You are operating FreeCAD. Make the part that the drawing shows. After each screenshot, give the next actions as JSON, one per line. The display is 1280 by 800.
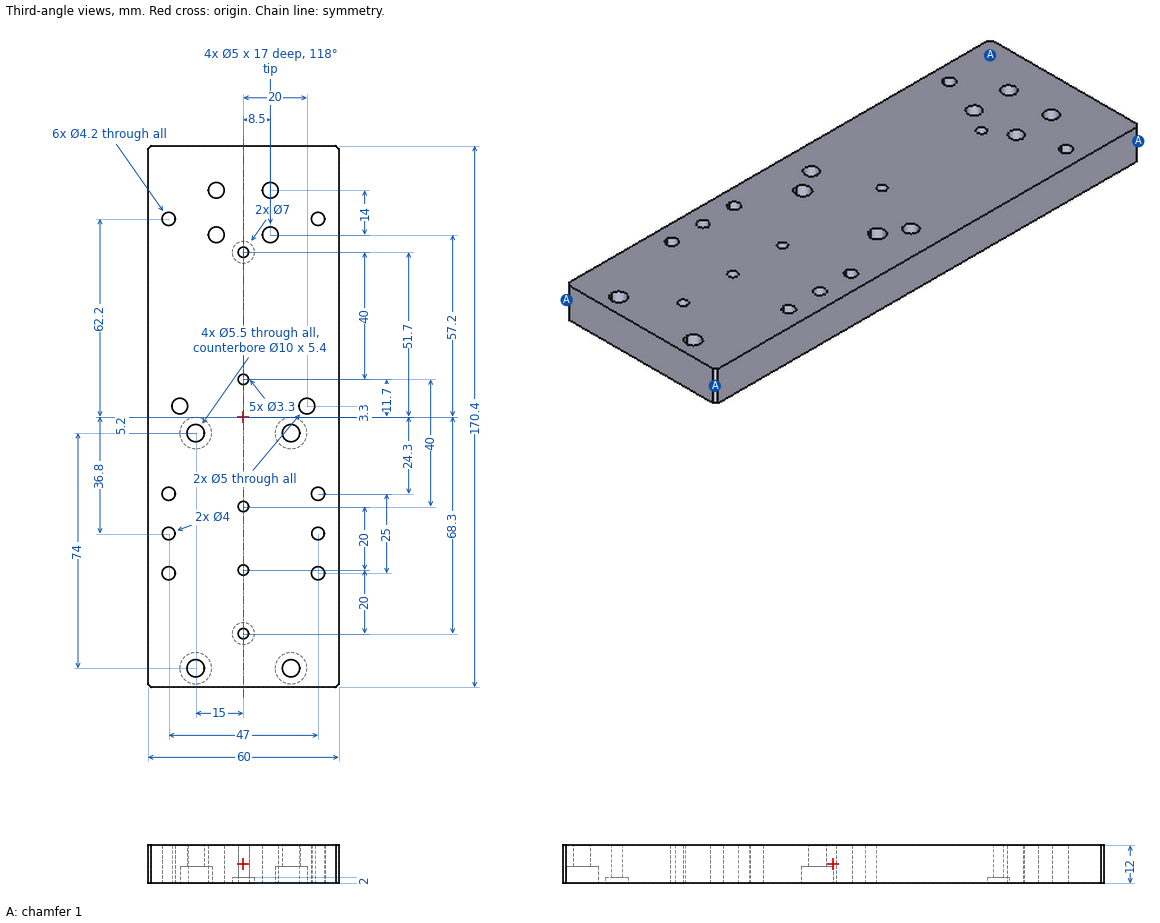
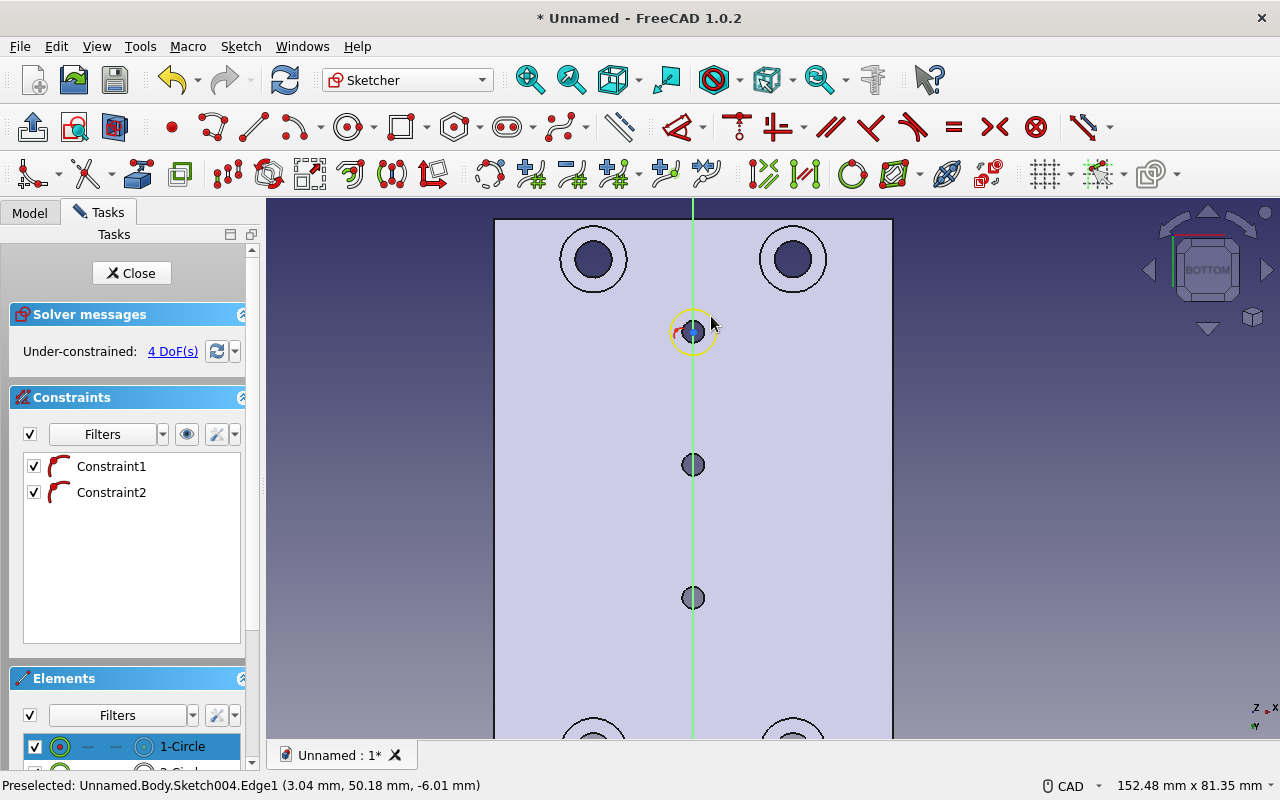
{"action": "left_click", "coordinate": [709, 316]}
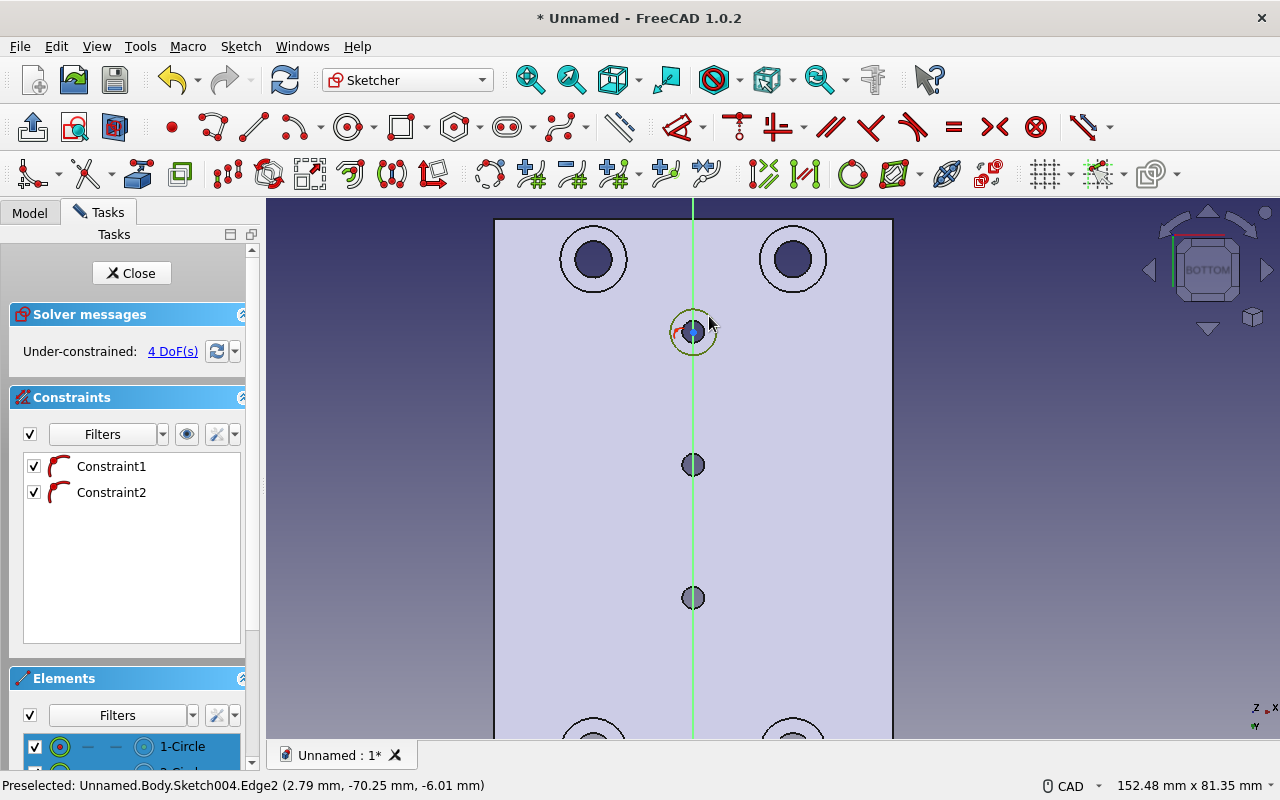
{"action": "key", "text": "e"}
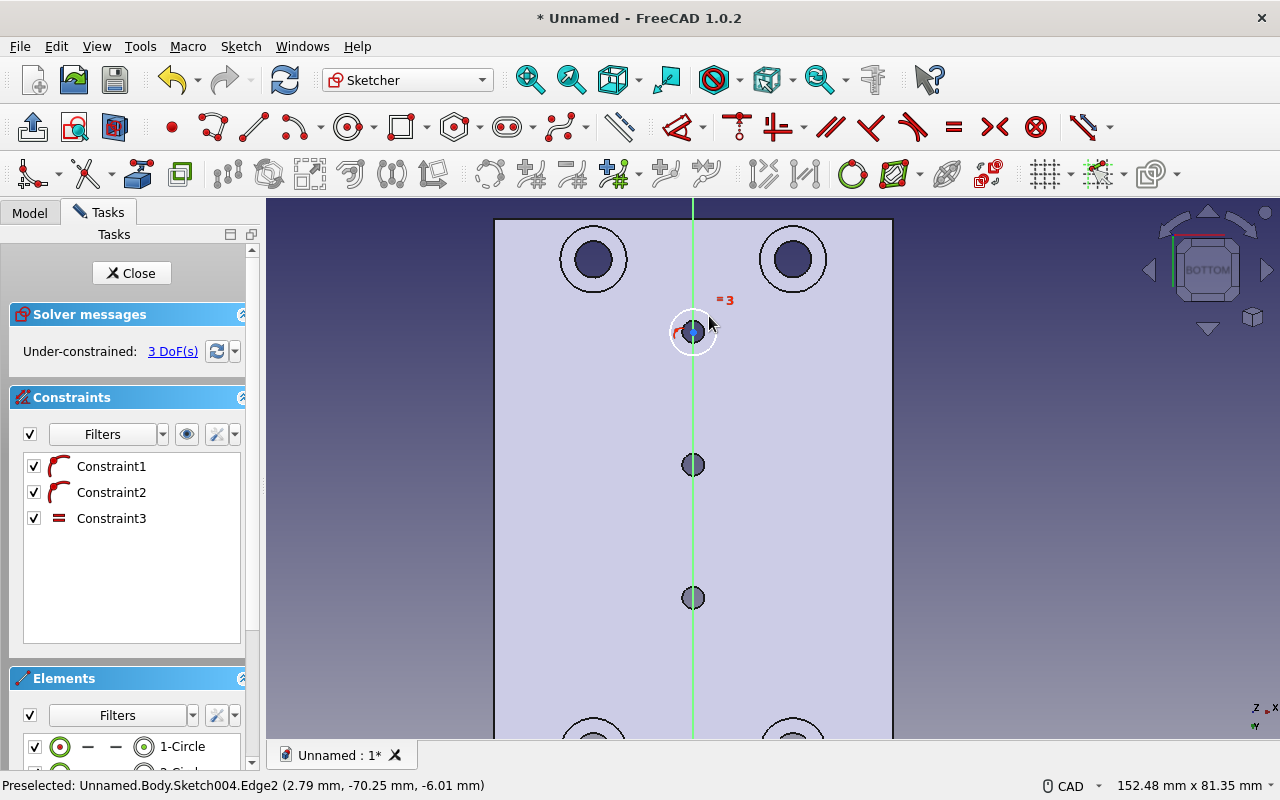
{"action": "left_click", "coordinate": [676, 128]}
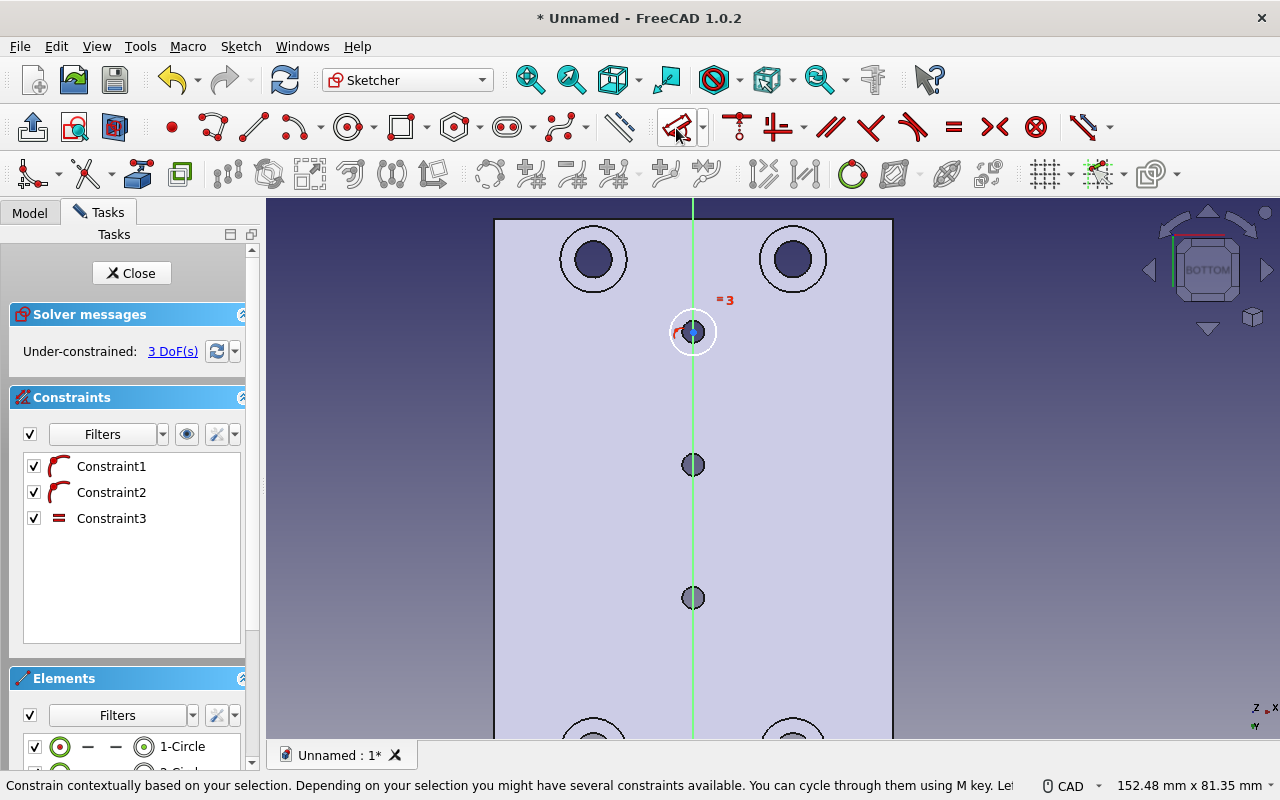
{"action": "scroll", "coordinate": [711, 316], "scroll_direction": "down", "scroll_amount": 5}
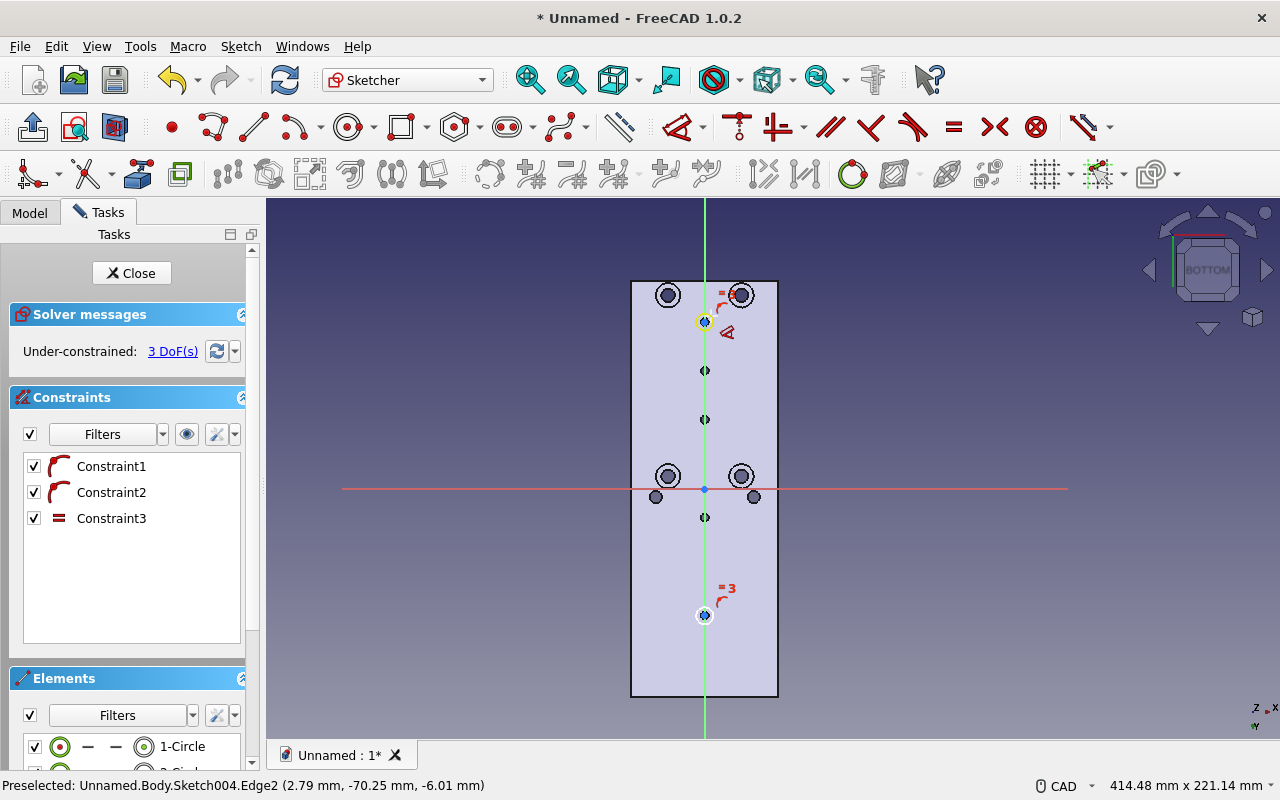
{"action": "scroll", "coordinate": [711, 610], "scroll_direction": "up", "scroll_amount": 5}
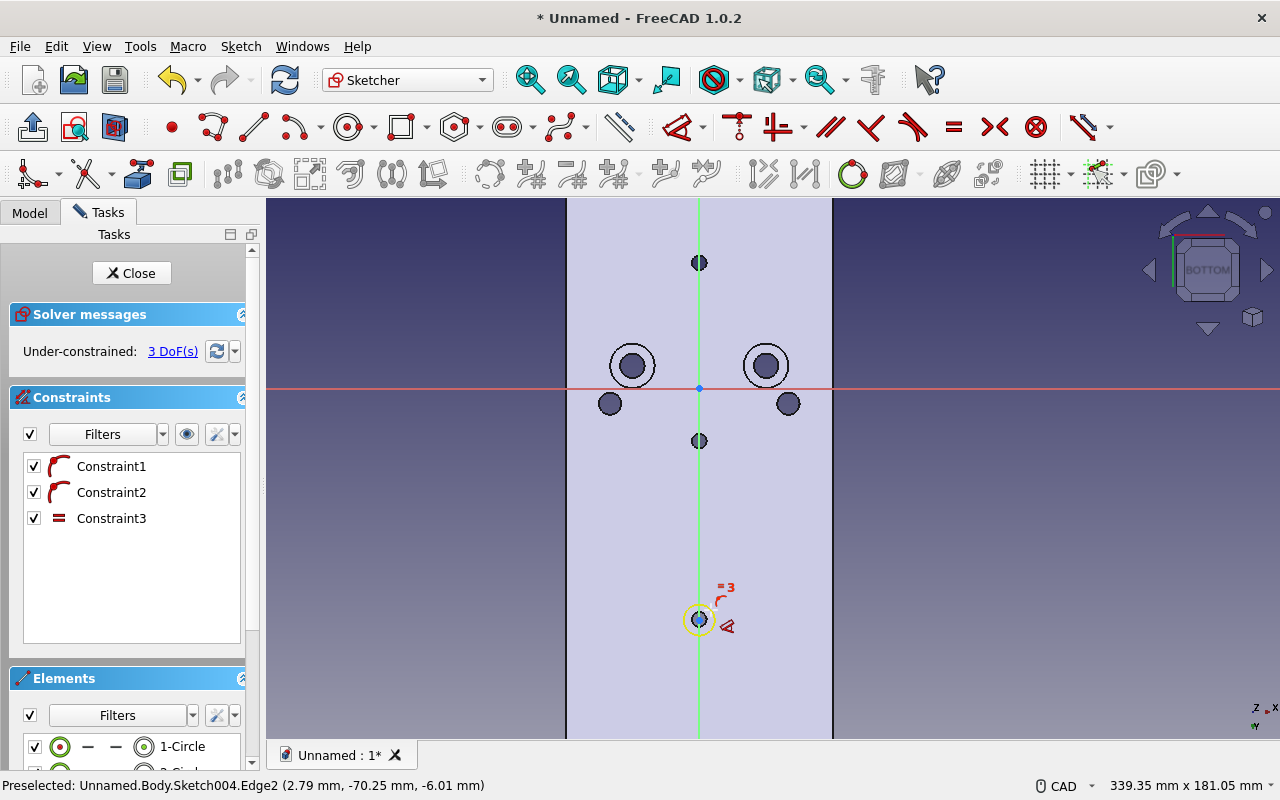
{"action": "left_click", "coordinate": [710, 608]}
{"action": "left_click", "coordinate": [733, 585]}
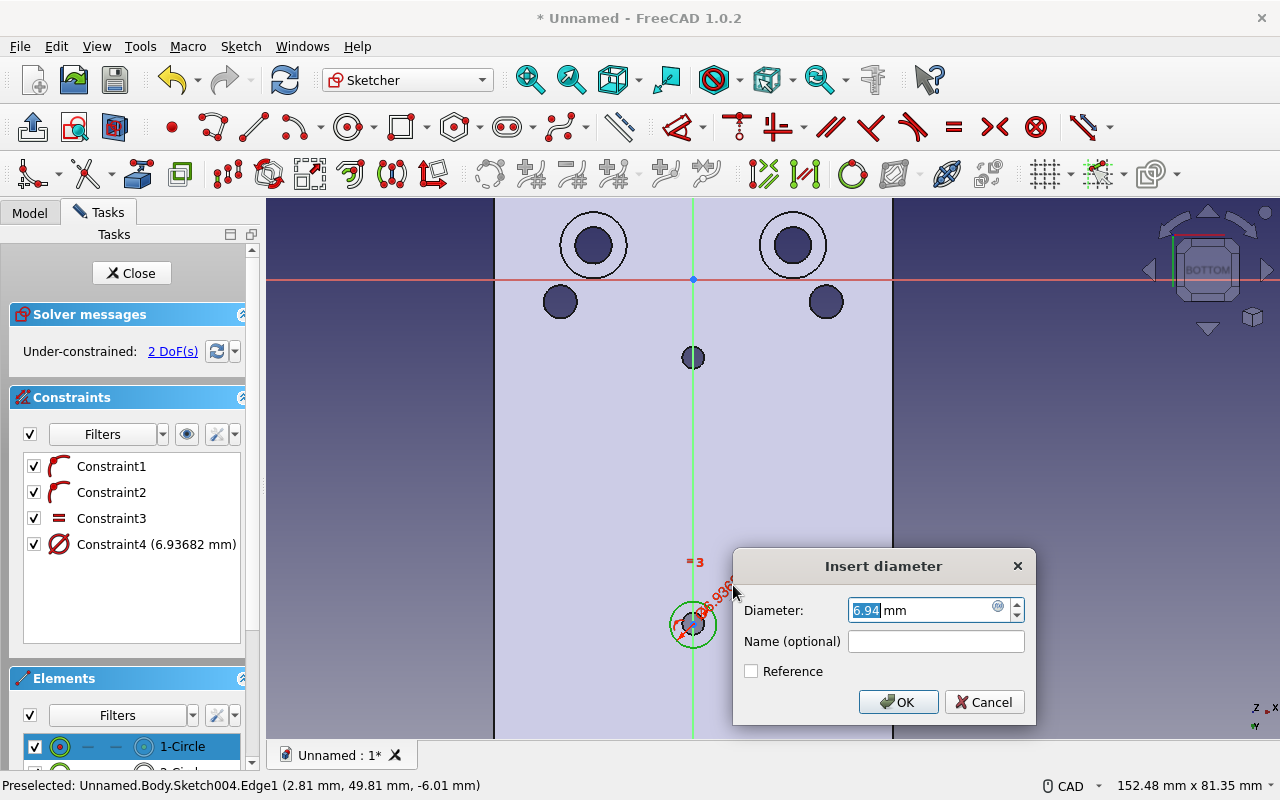
{"action": "type", "text": "7"}
{"action": "key", "text": "Return"}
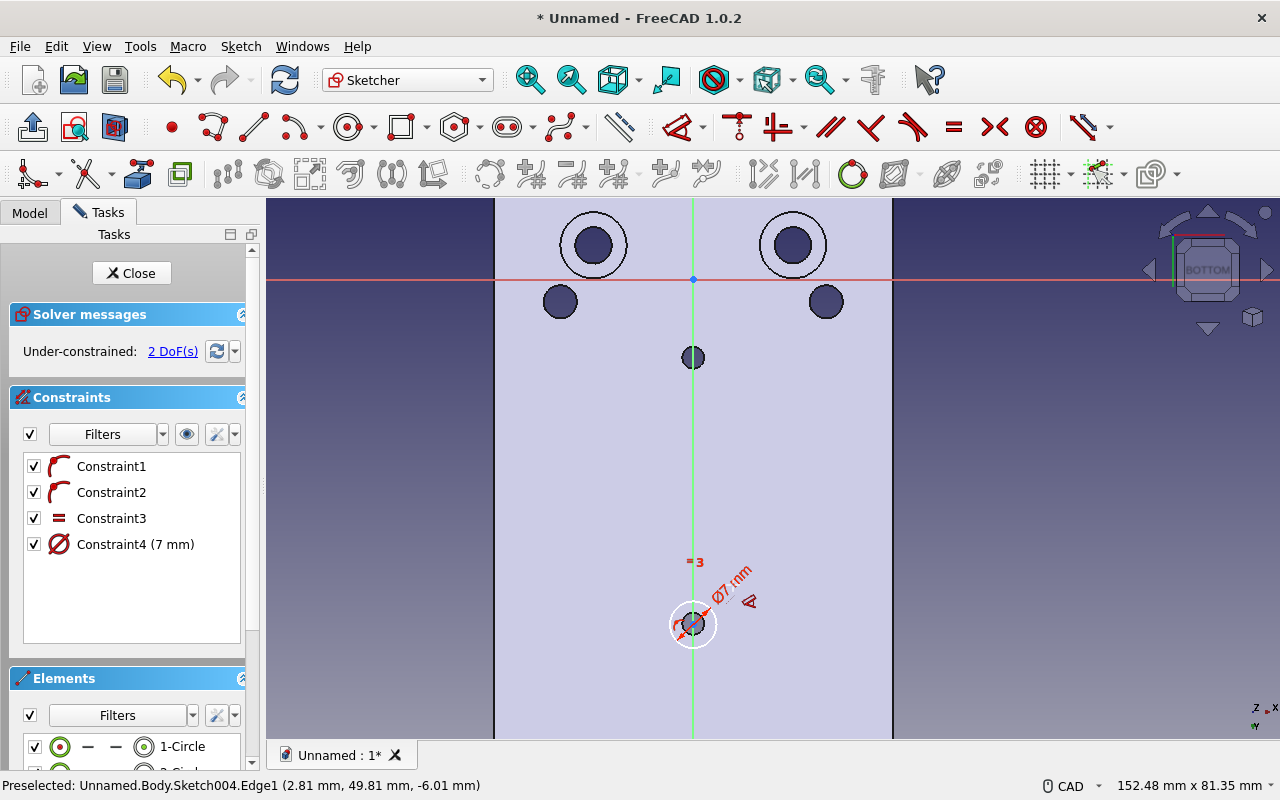
{"action": "left_click", "coordinate": [693, 625]}
{"action": "left_click", "coordinate": [727, 452]}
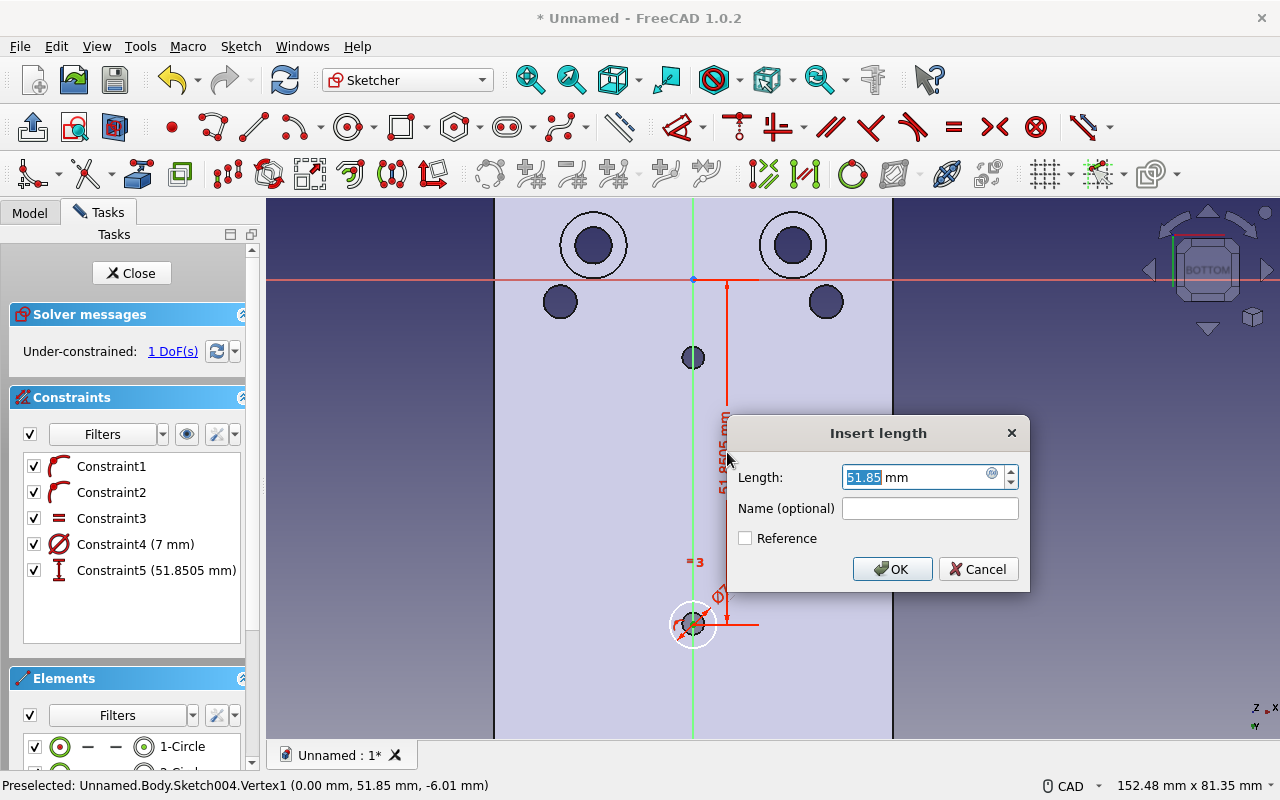
{"action": "type", "text": "51.7"}
{"action": "key", "text": "Return"}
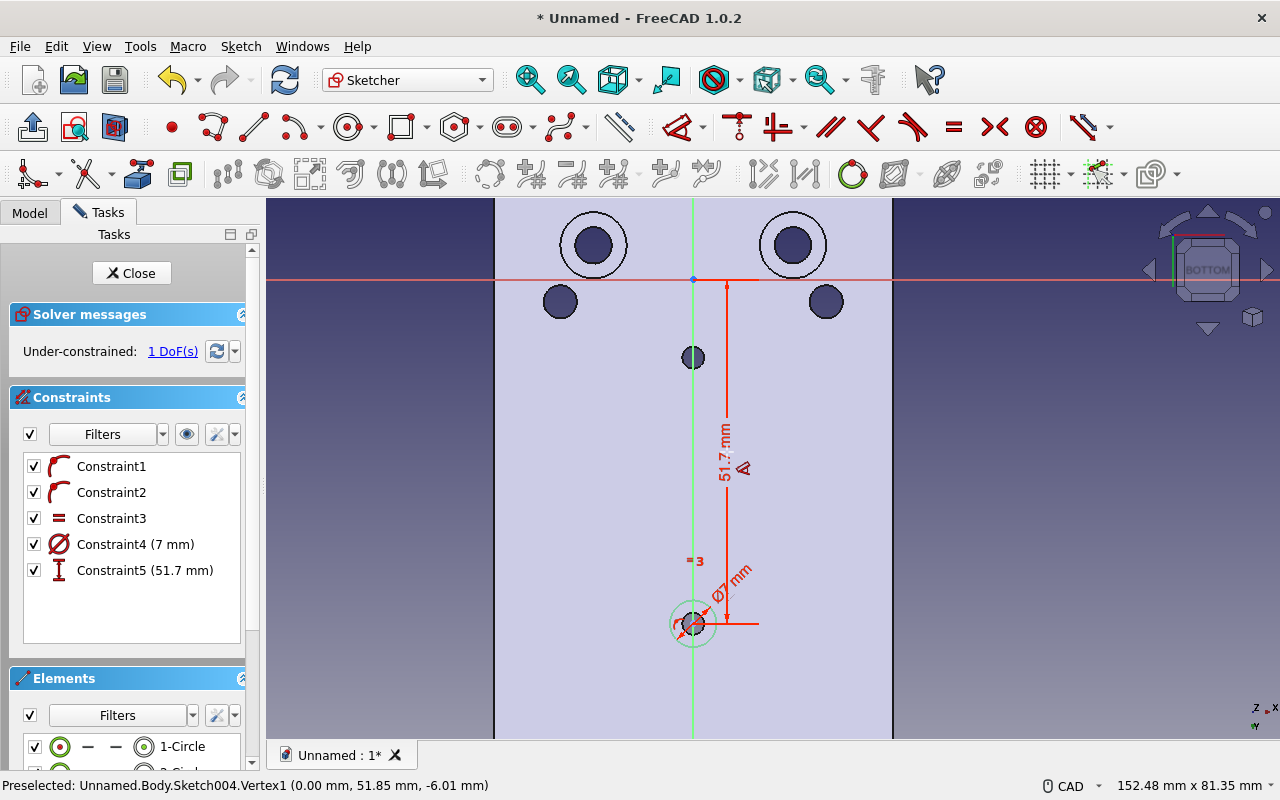
{"action": "scroll", "coordinate": [711, 610], "scroll_direction": "down", "scroll_amount": 5}